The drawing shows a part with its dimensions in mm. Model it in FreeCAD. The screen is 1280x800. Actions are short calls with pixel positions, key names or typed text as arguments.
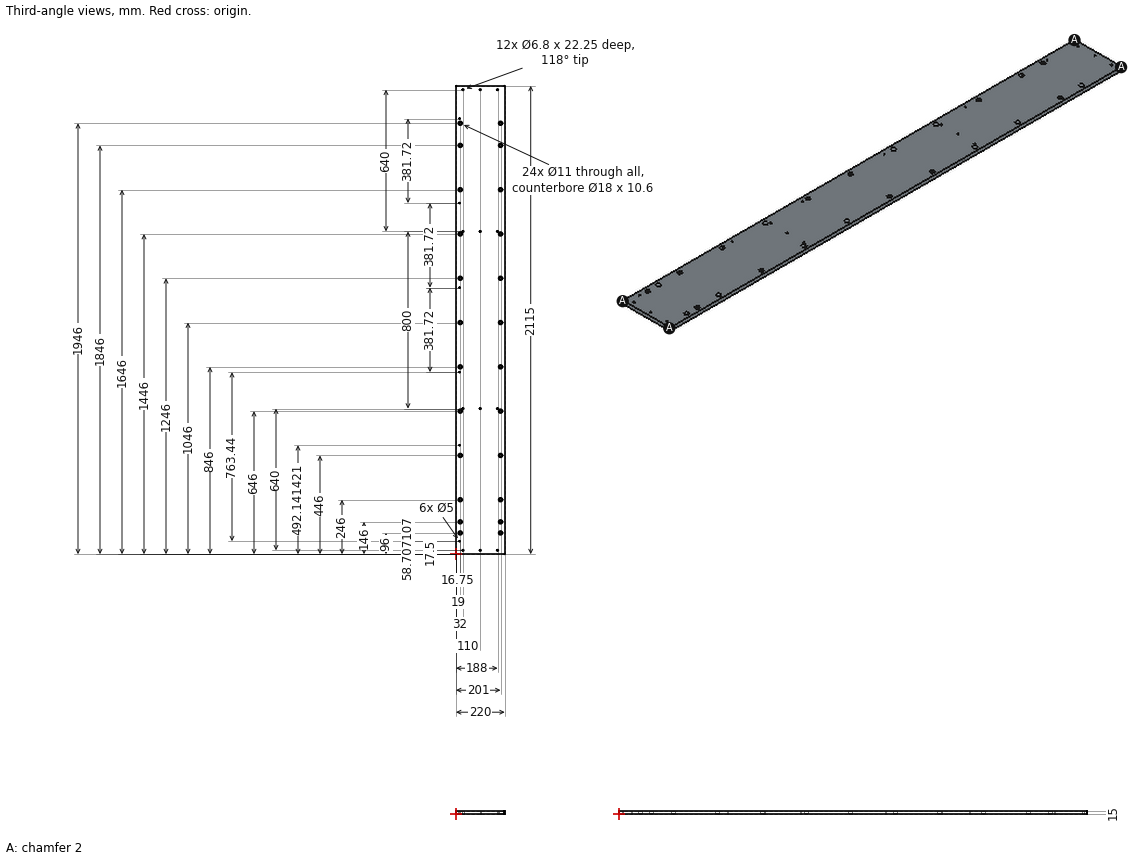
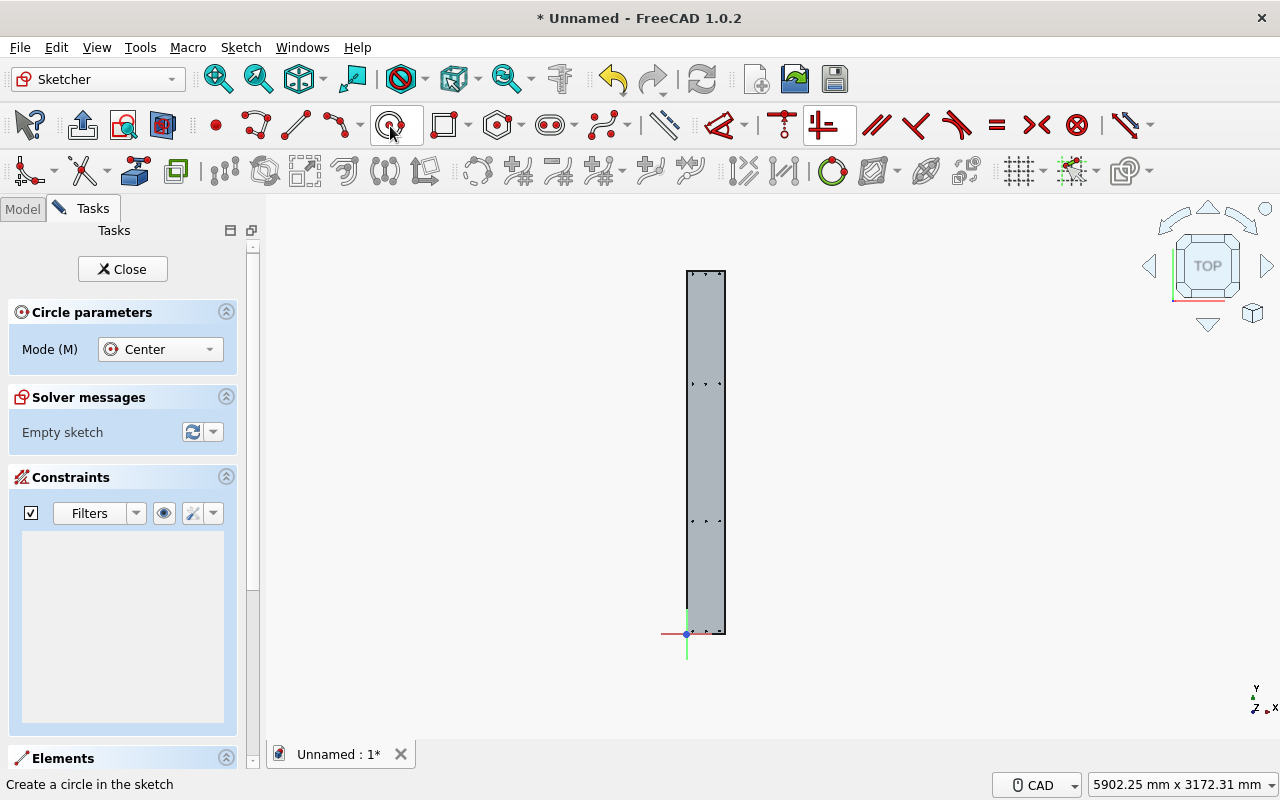
scroll(690, 300, up, 16)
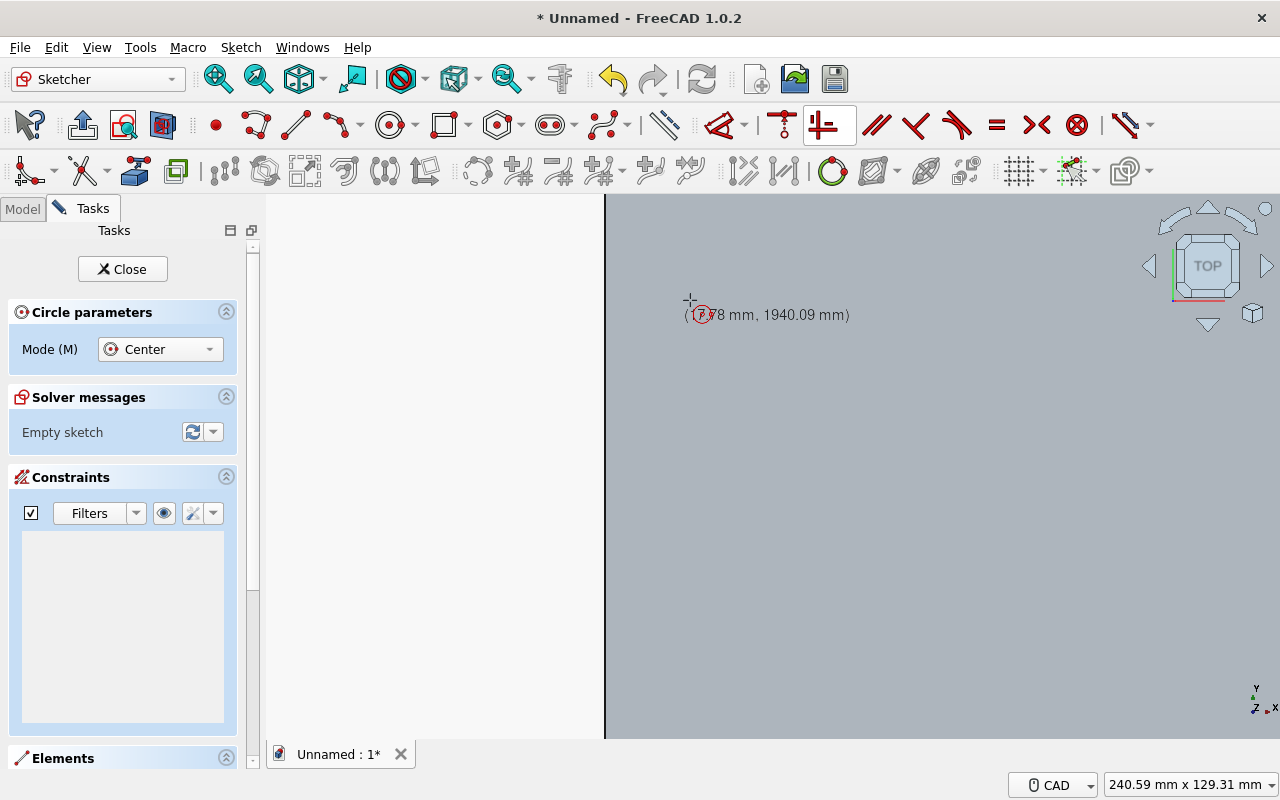
scroll(687, 261, down, 15)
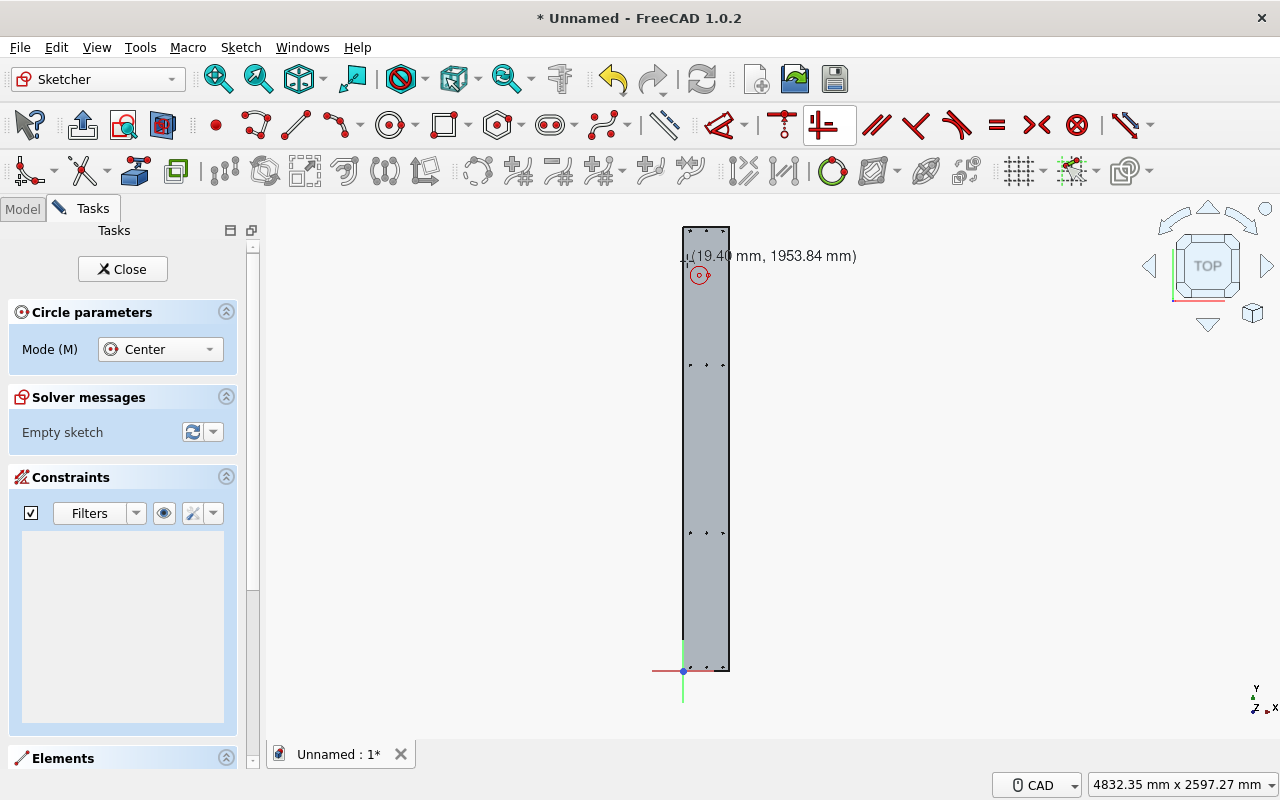
scroll(687, 263, up, 7)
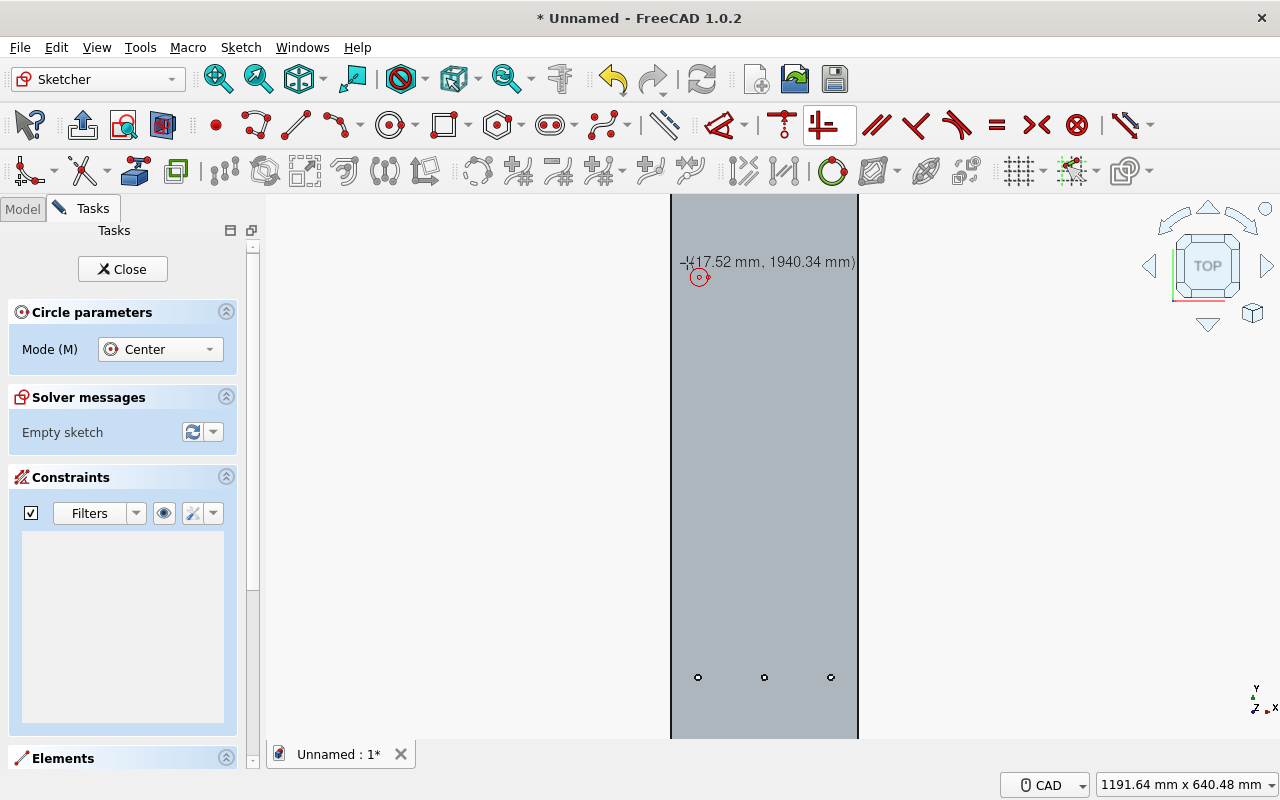
click(687, 262)
move(690, 259)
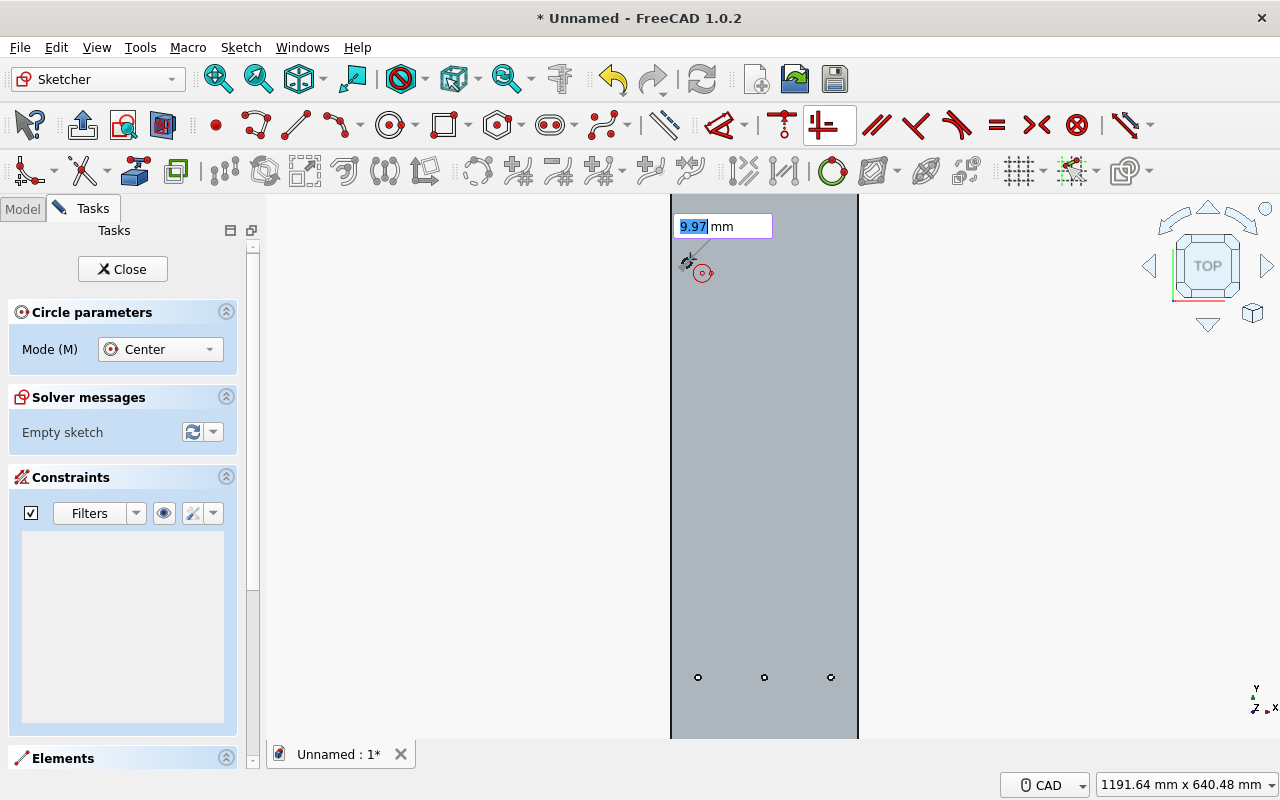
text(11)
key(Return)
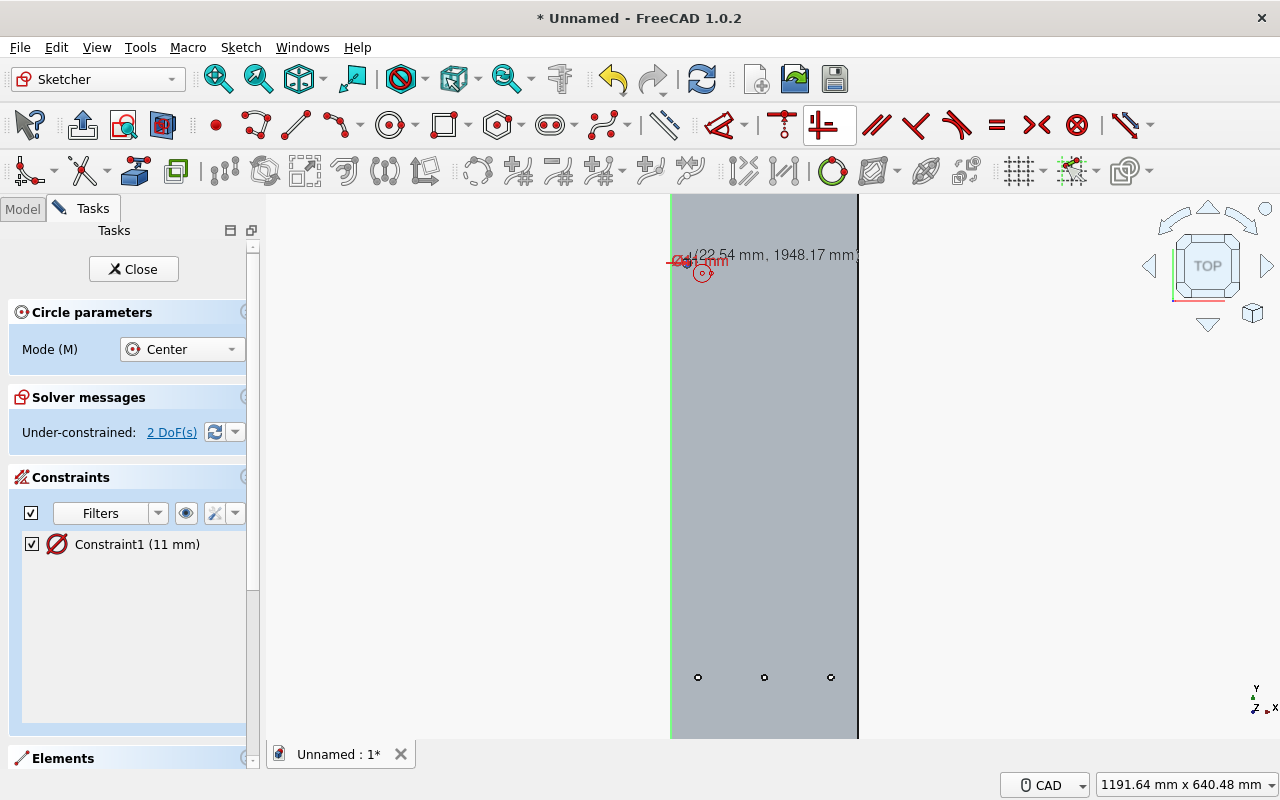
scroll(842, 262, up, 8)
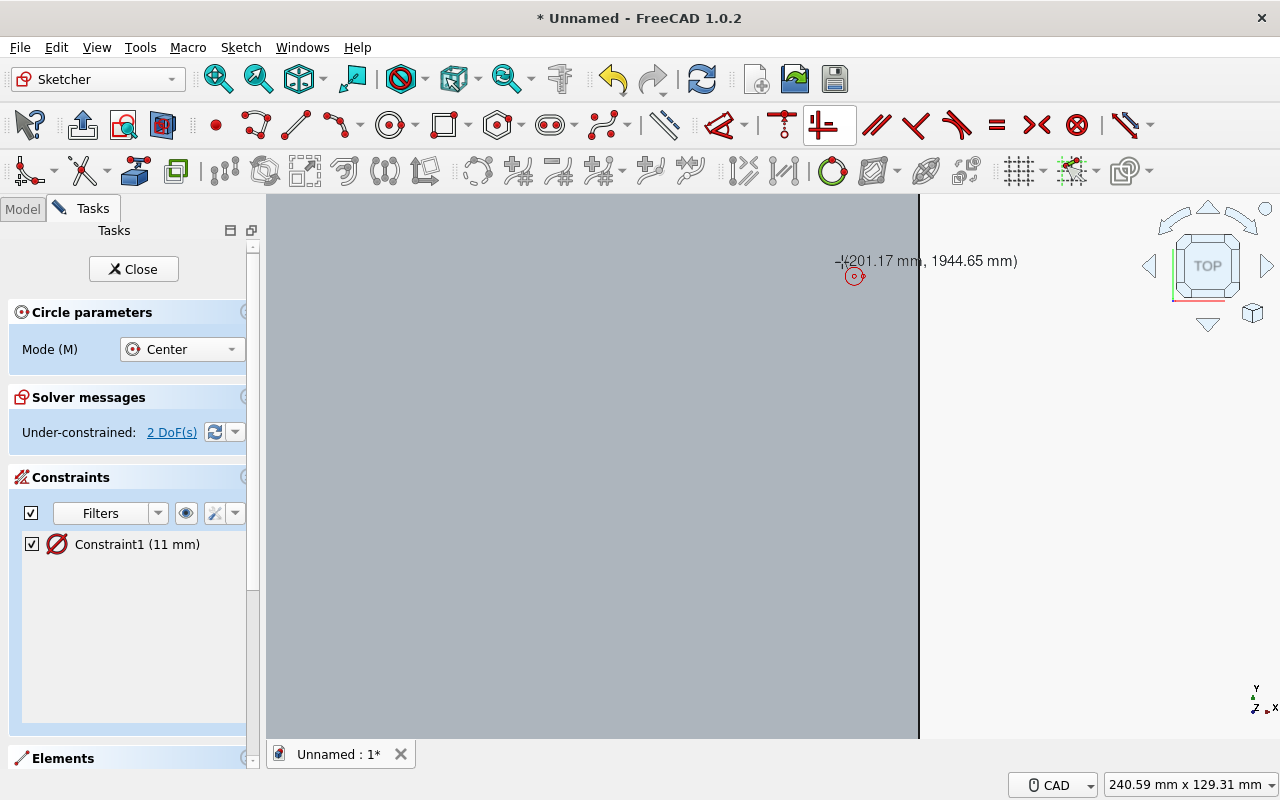
scroll(719, 263, down, 15)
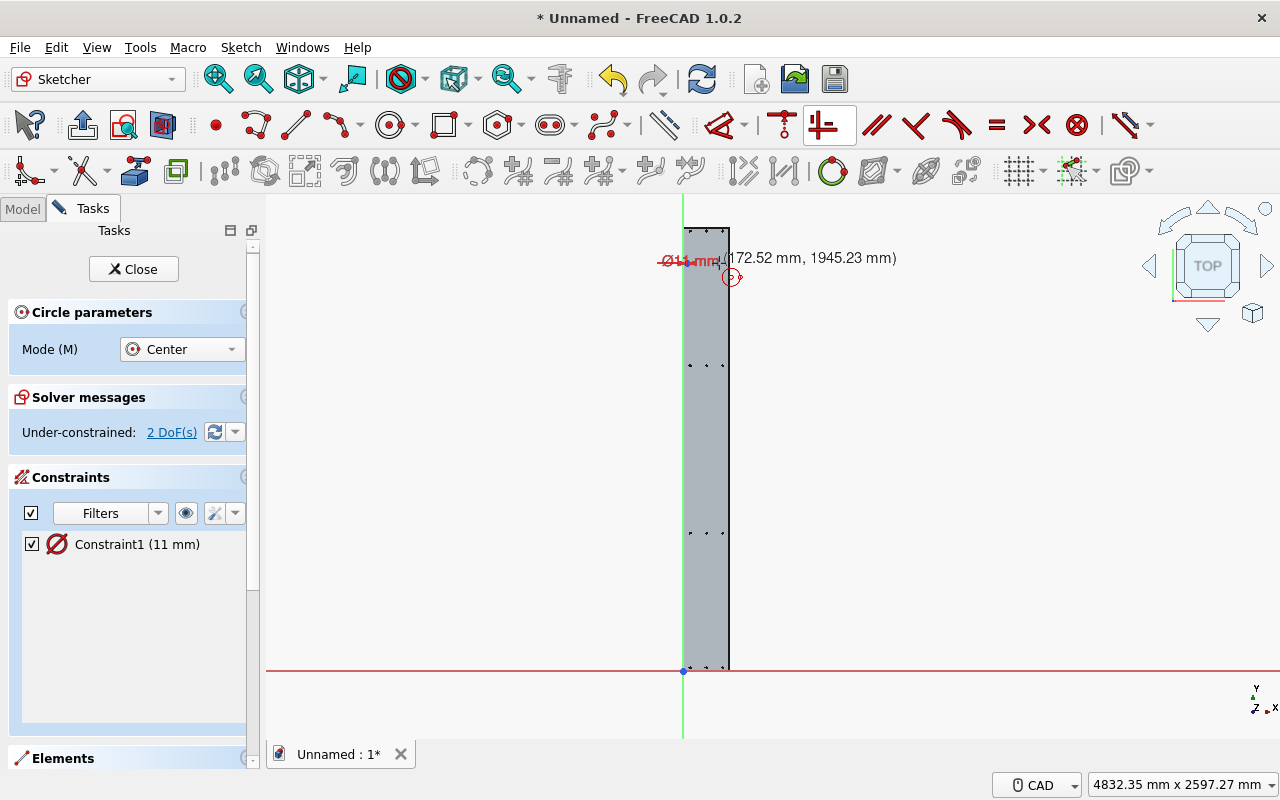
click(725, 263)
move(726, 262)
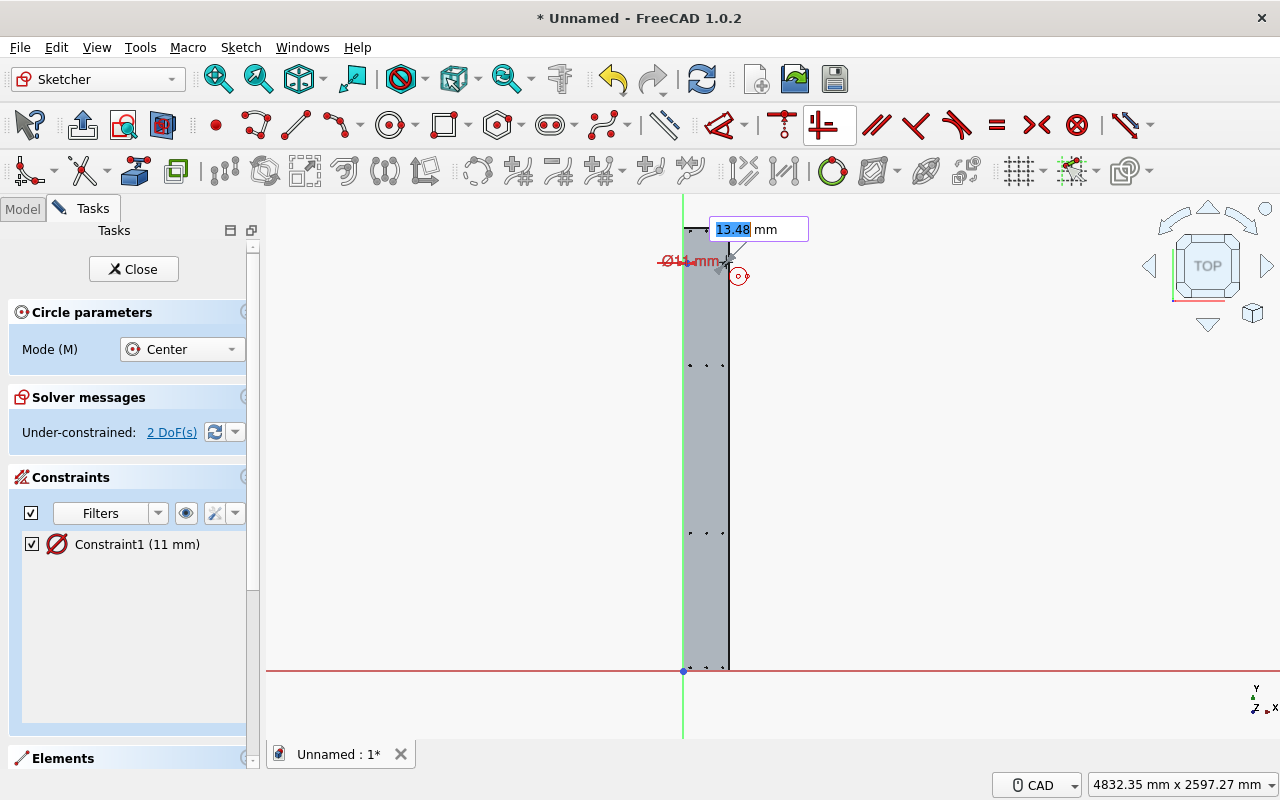
text(11)
key(Return)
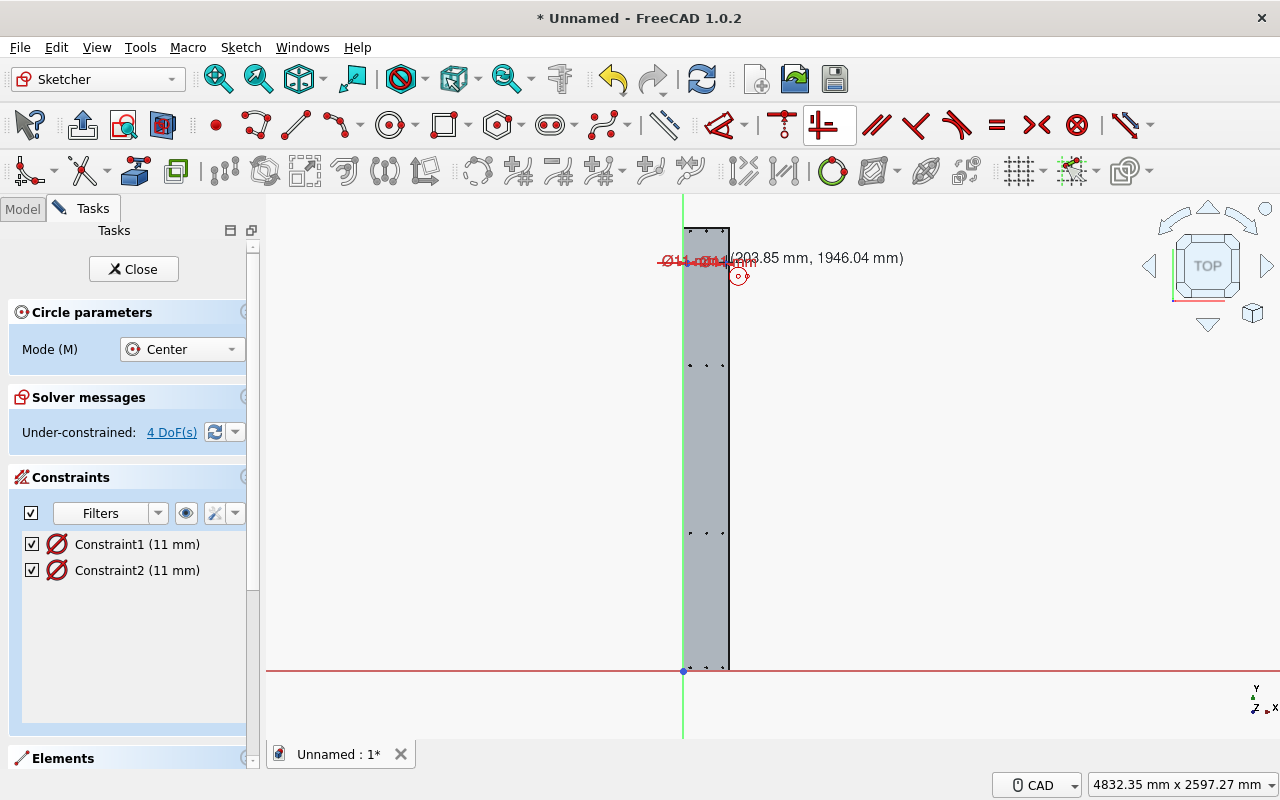
scroll(687, 284, up, 15)